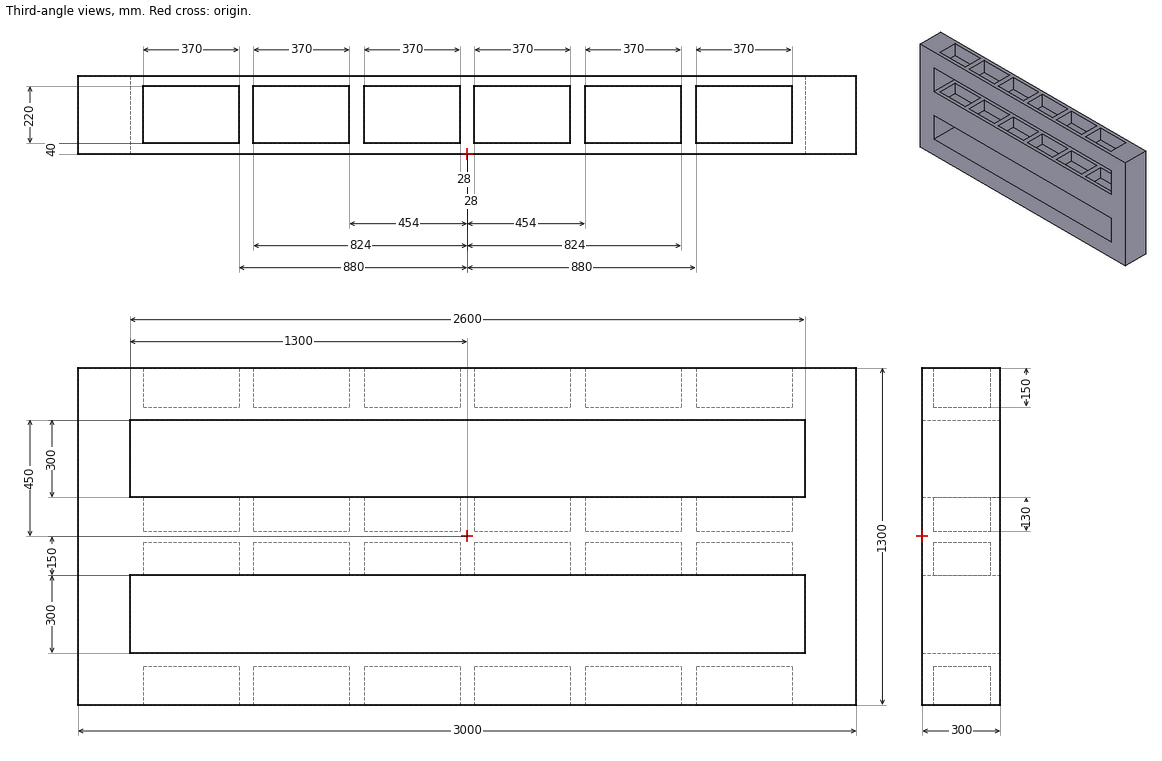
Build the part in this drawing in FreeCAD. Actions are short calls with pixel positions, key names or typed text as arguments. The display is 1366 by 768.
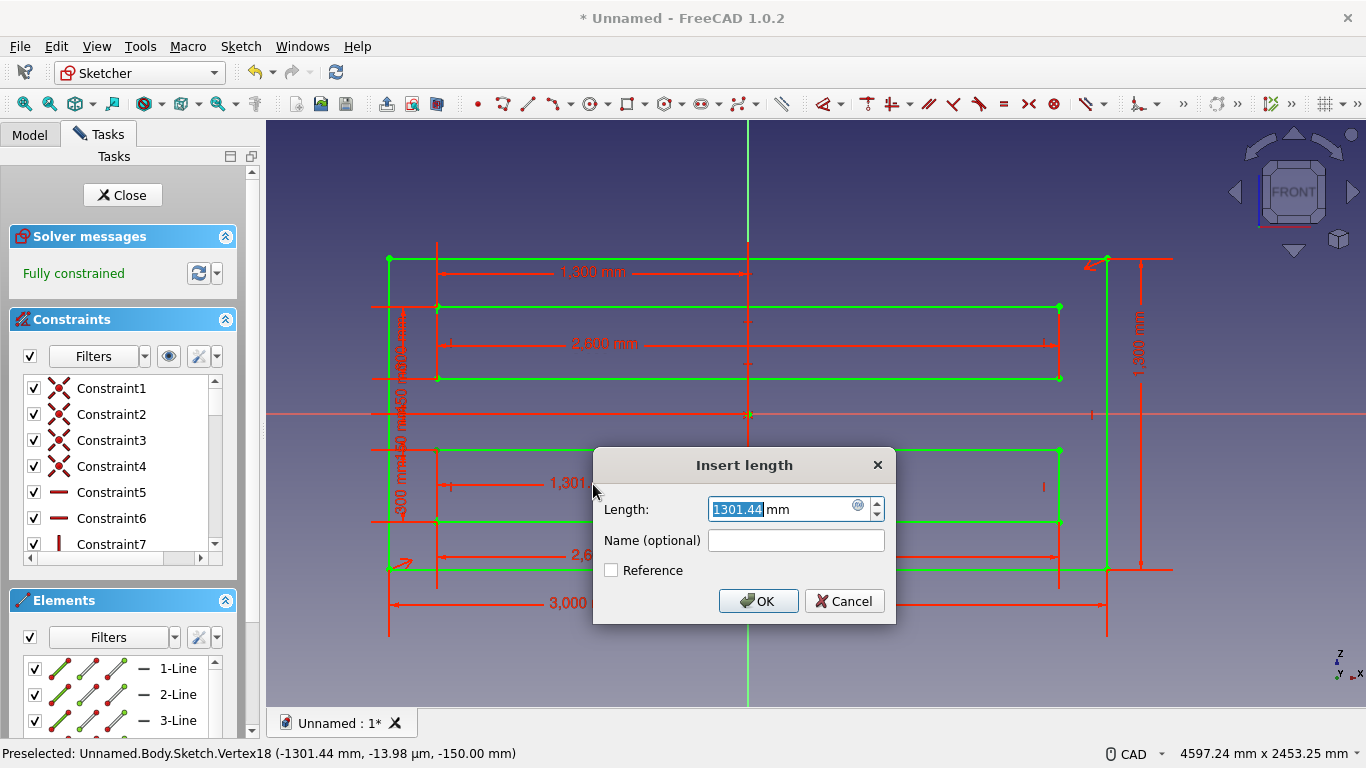
text(1300)
key(Return)
key(Escape)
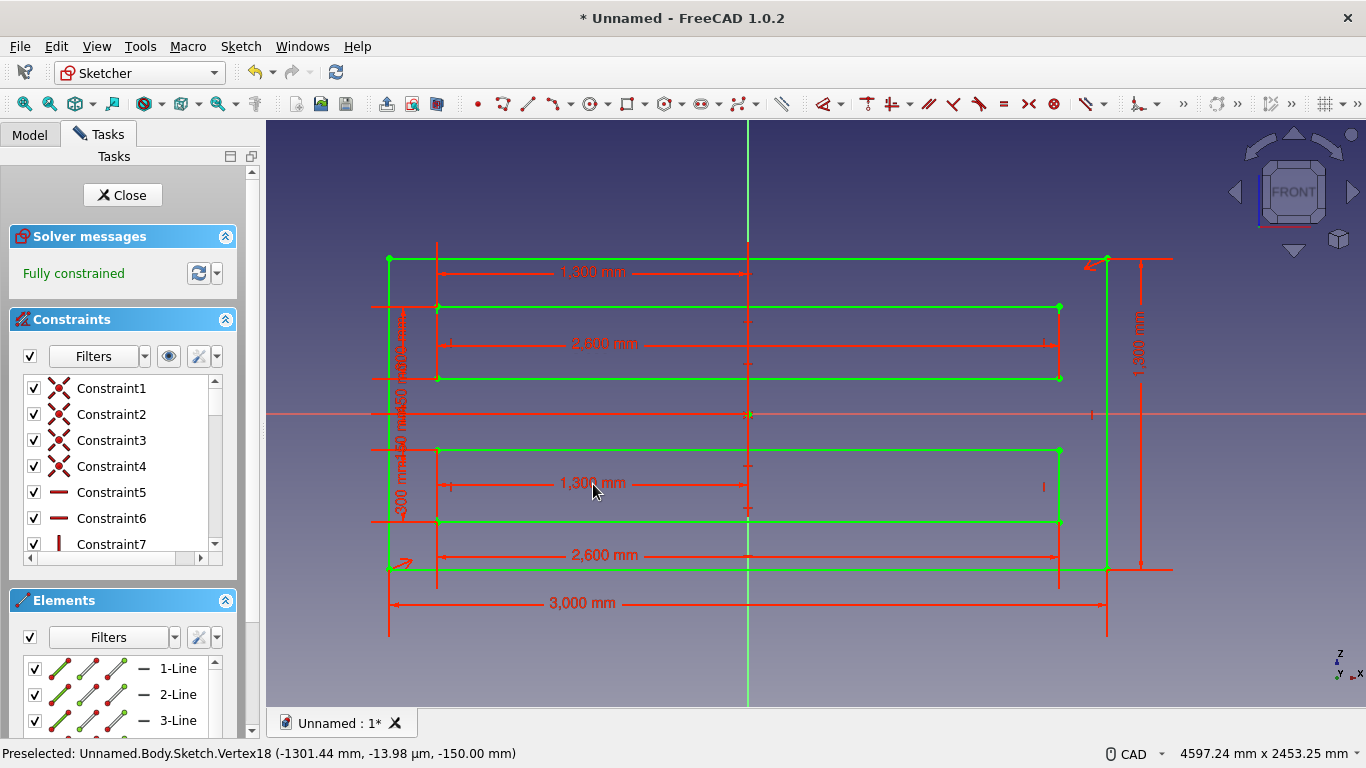
click(123, 195)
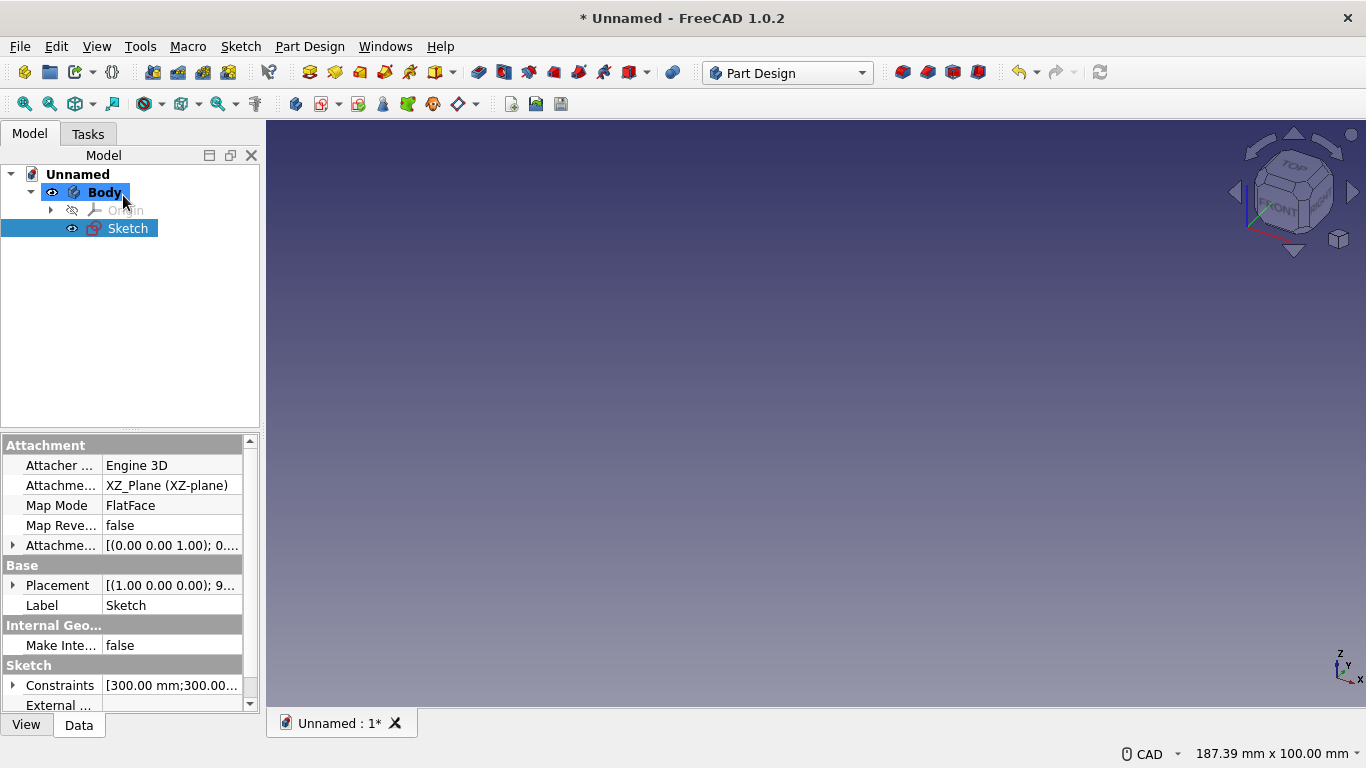
click(310, 72)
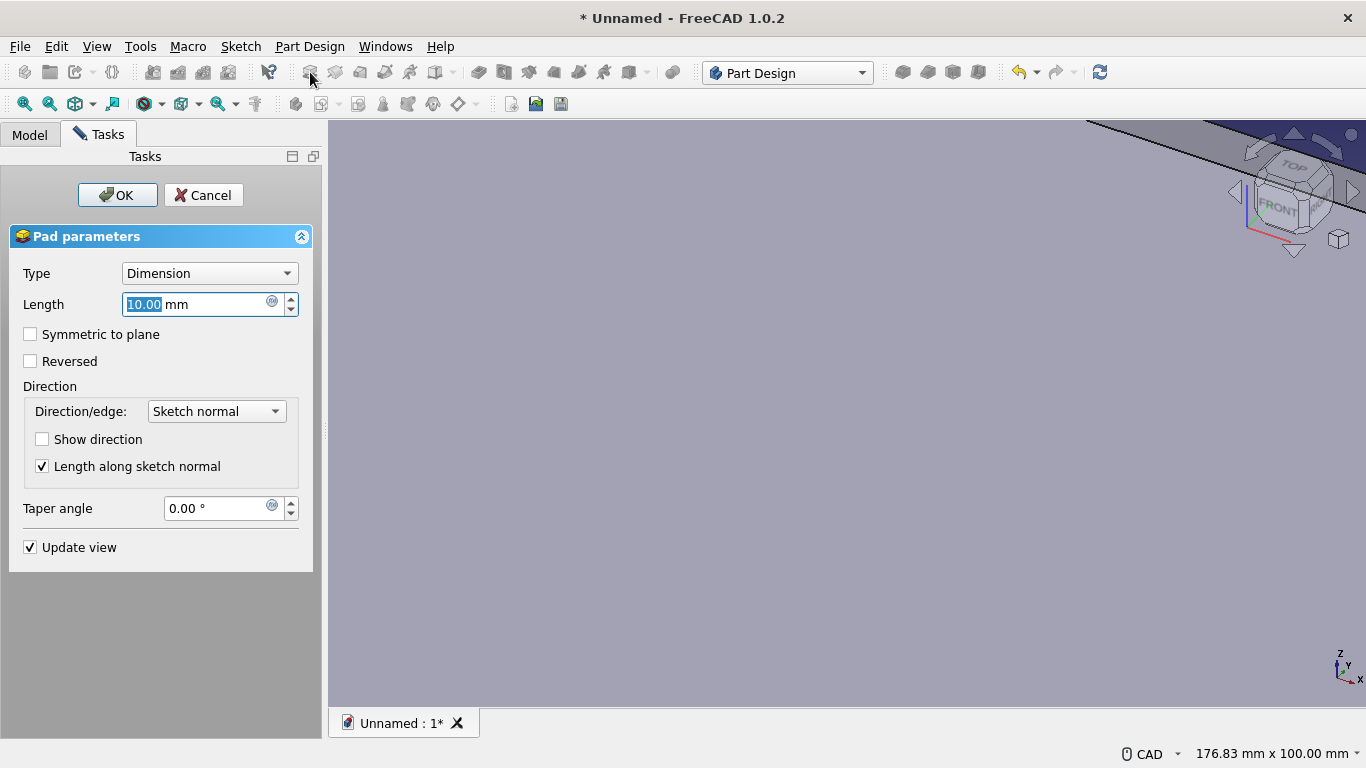
text(300)
key(Tab)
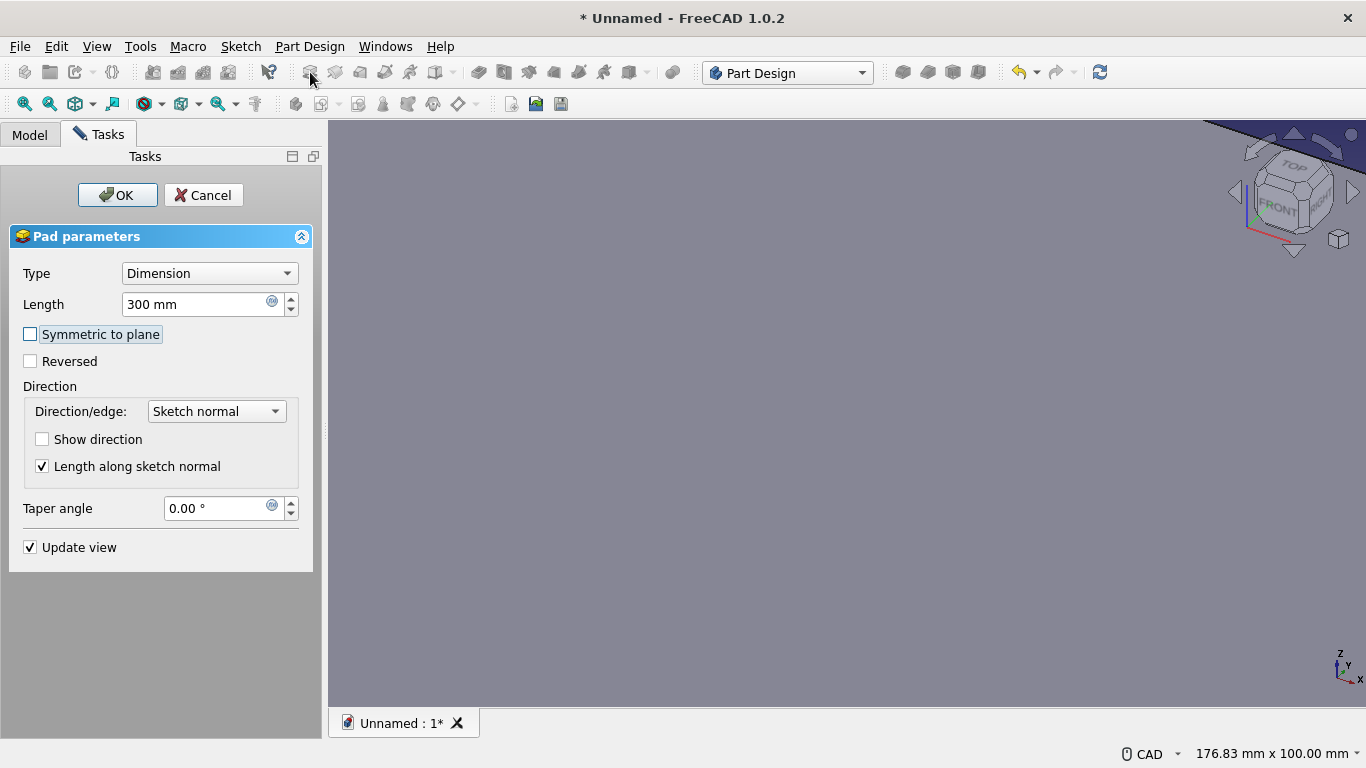
click(31, 361)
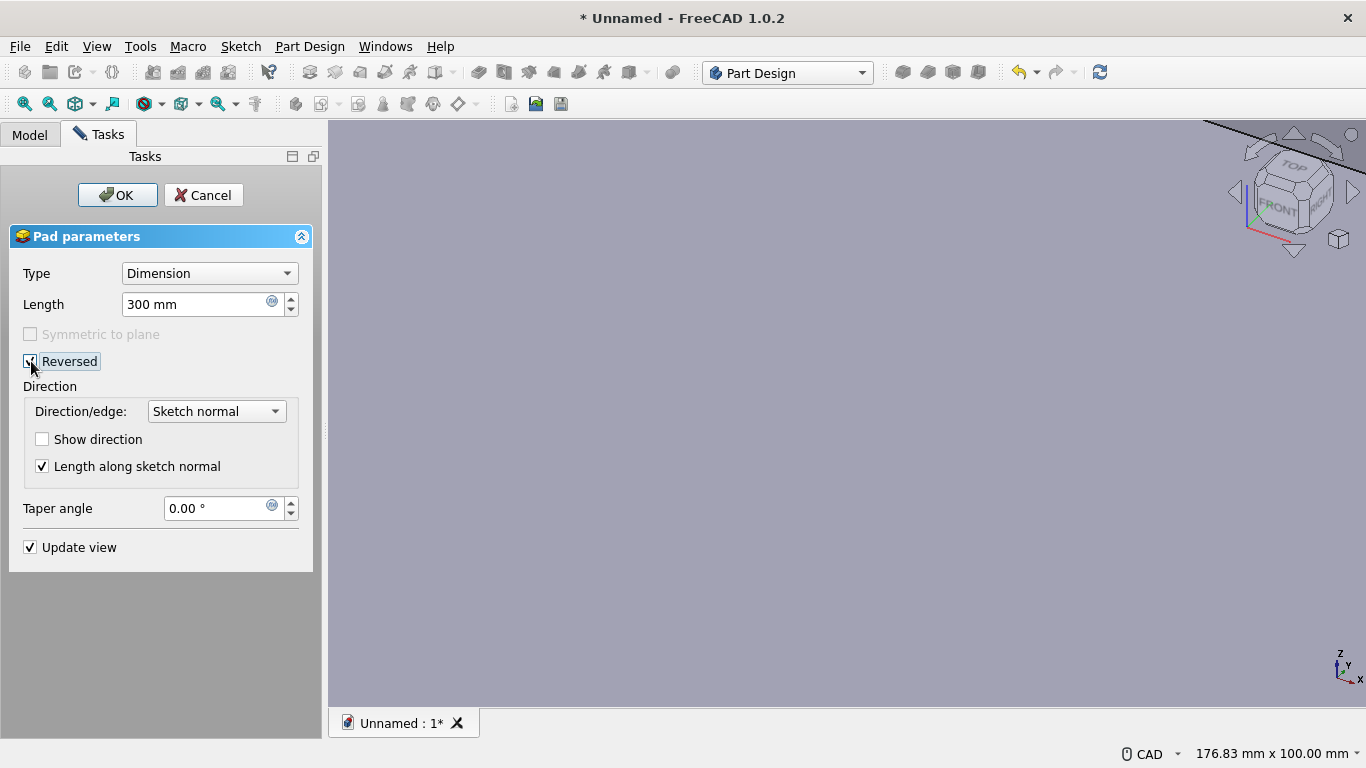
click(118, 195)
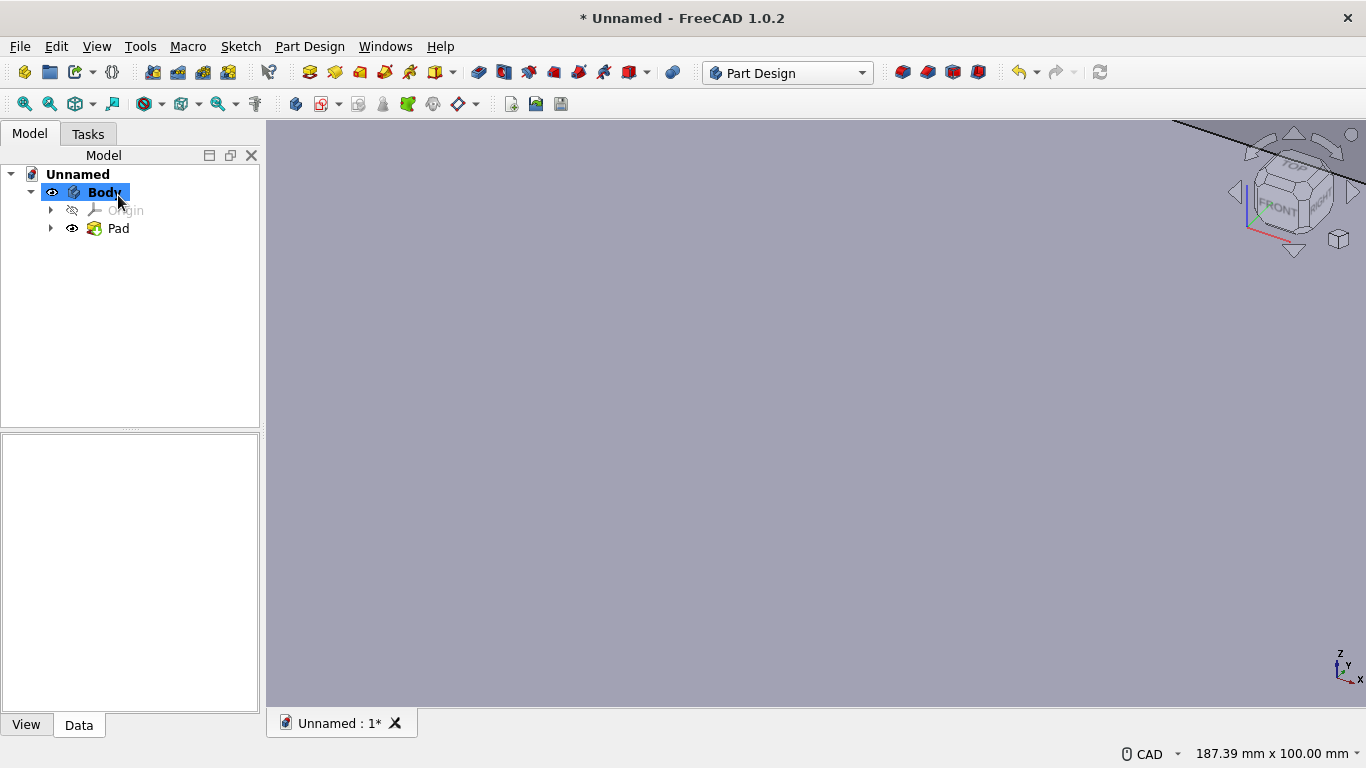
key(v)
key(f)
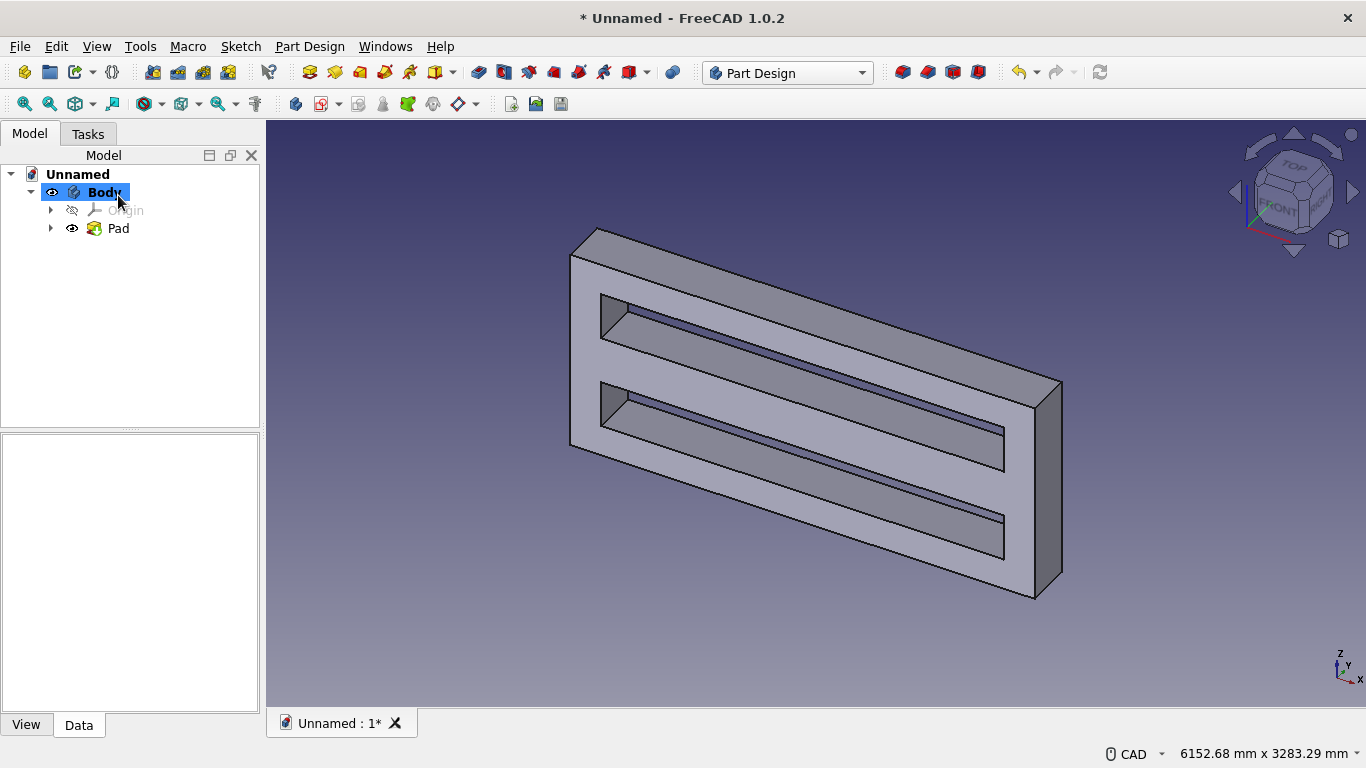
click(1015, 383)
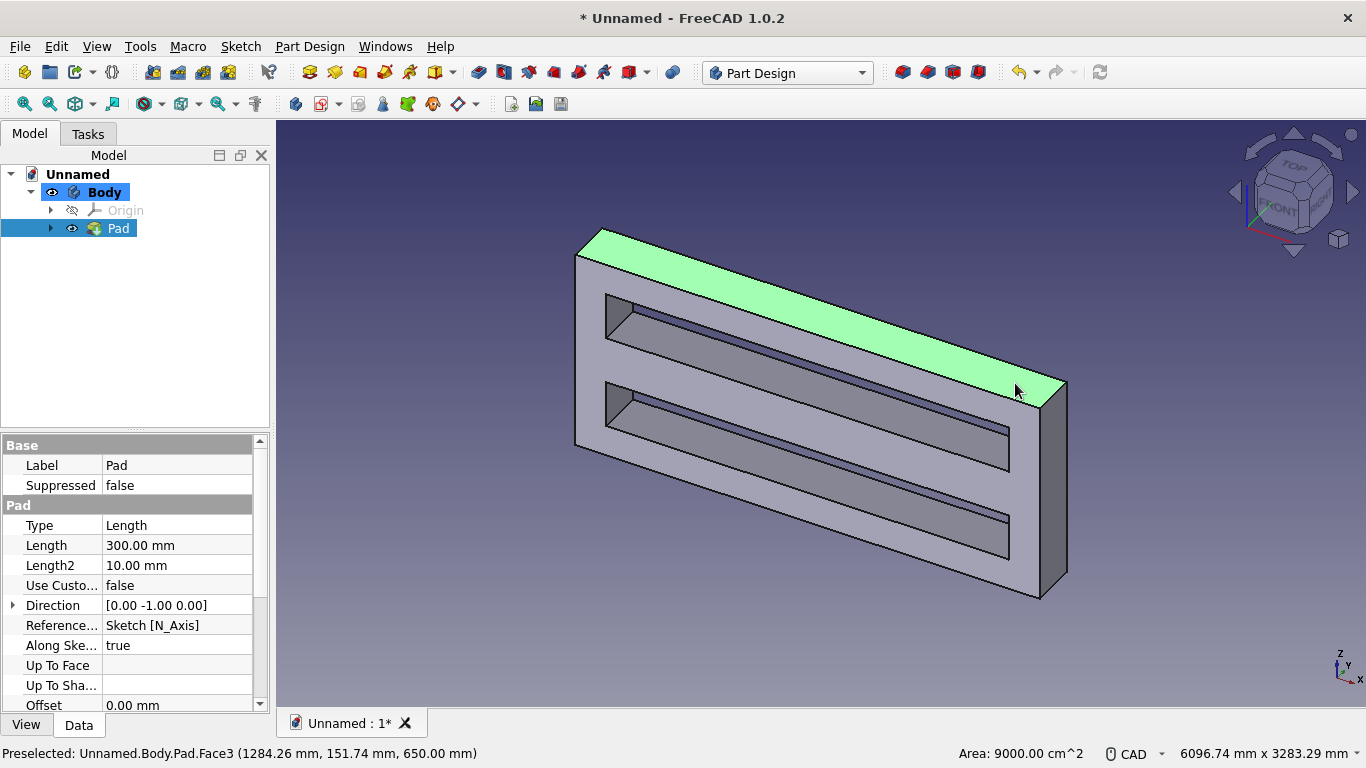
click(320, 104)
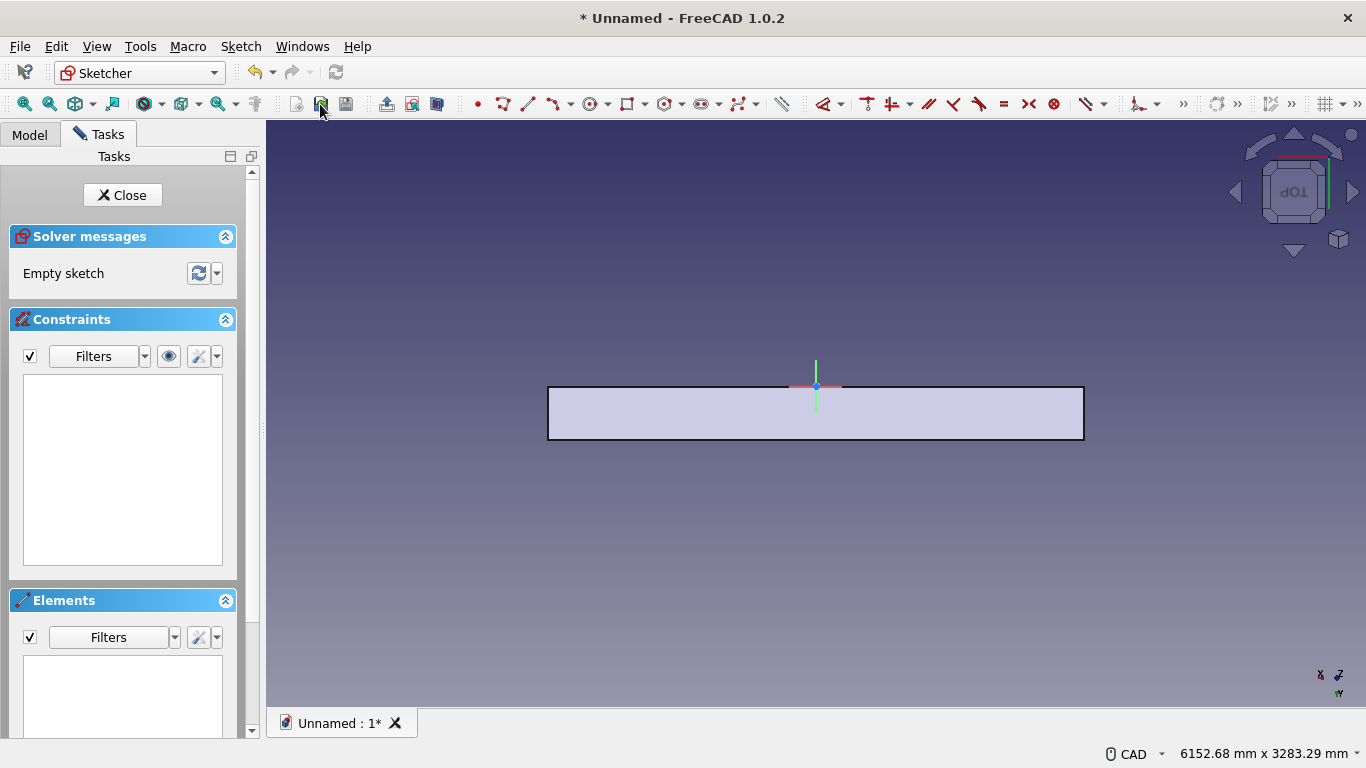
scroll(955, 403, up, 2)